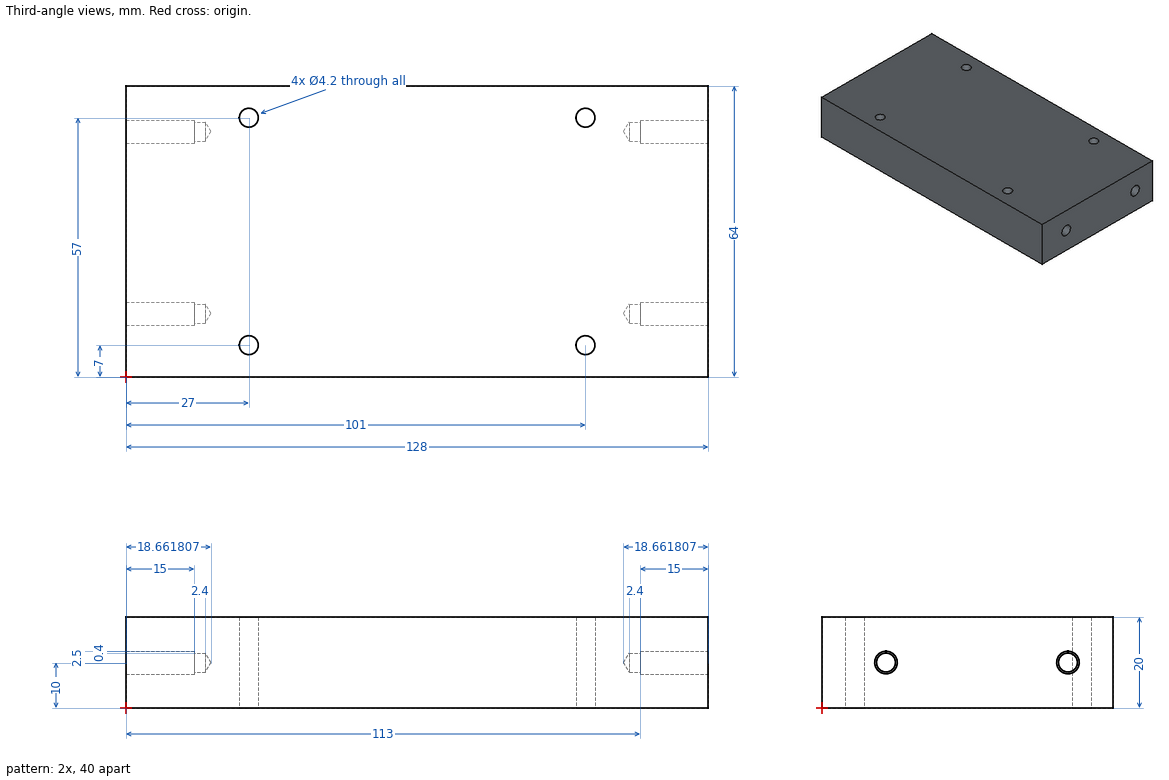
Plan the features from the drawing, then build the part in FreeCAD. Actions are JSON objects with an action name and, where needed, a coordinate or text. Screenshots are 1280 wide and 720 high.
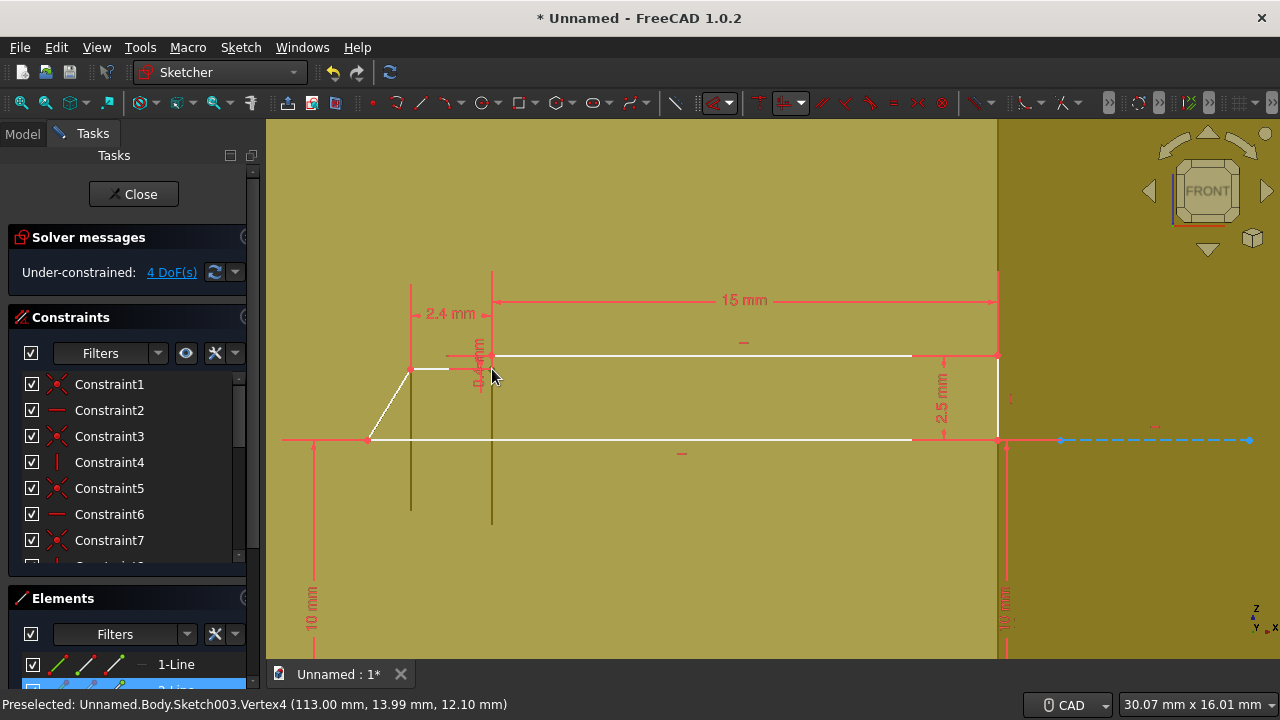
{"action": "key", "text": "l"}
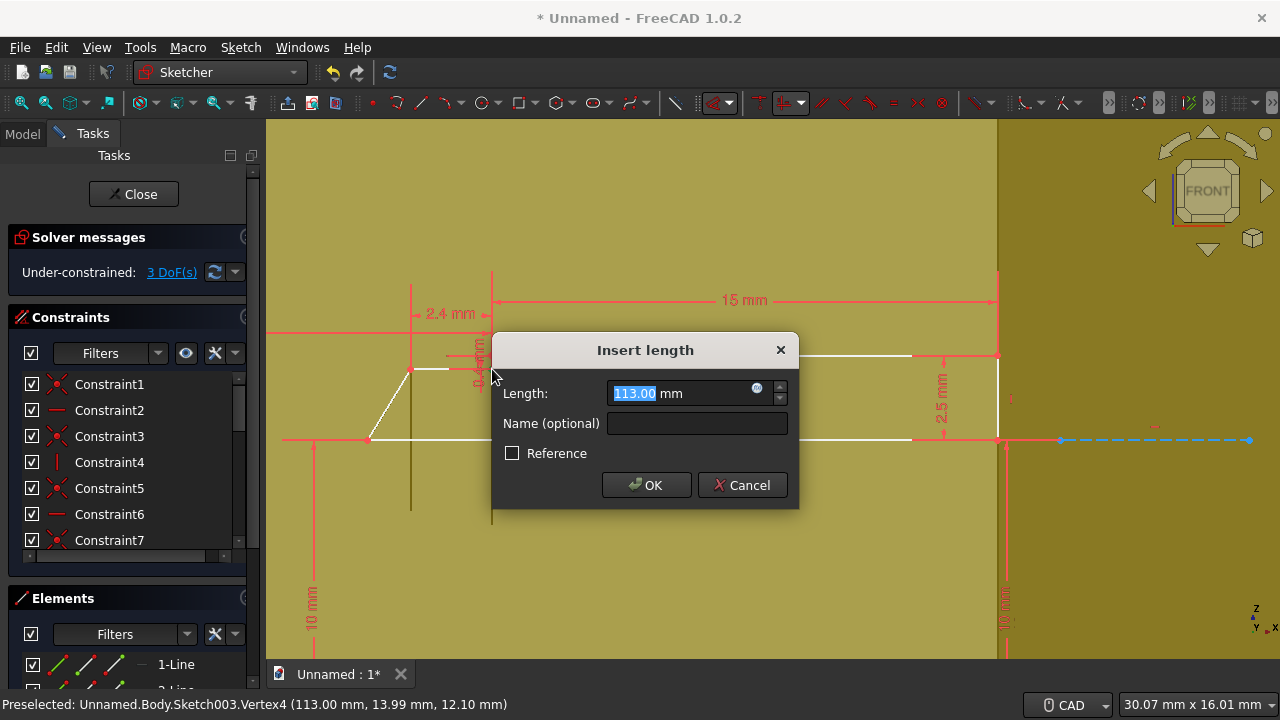
{"action": "type", "text": "113"}
{"action": "key", "text": "Return"}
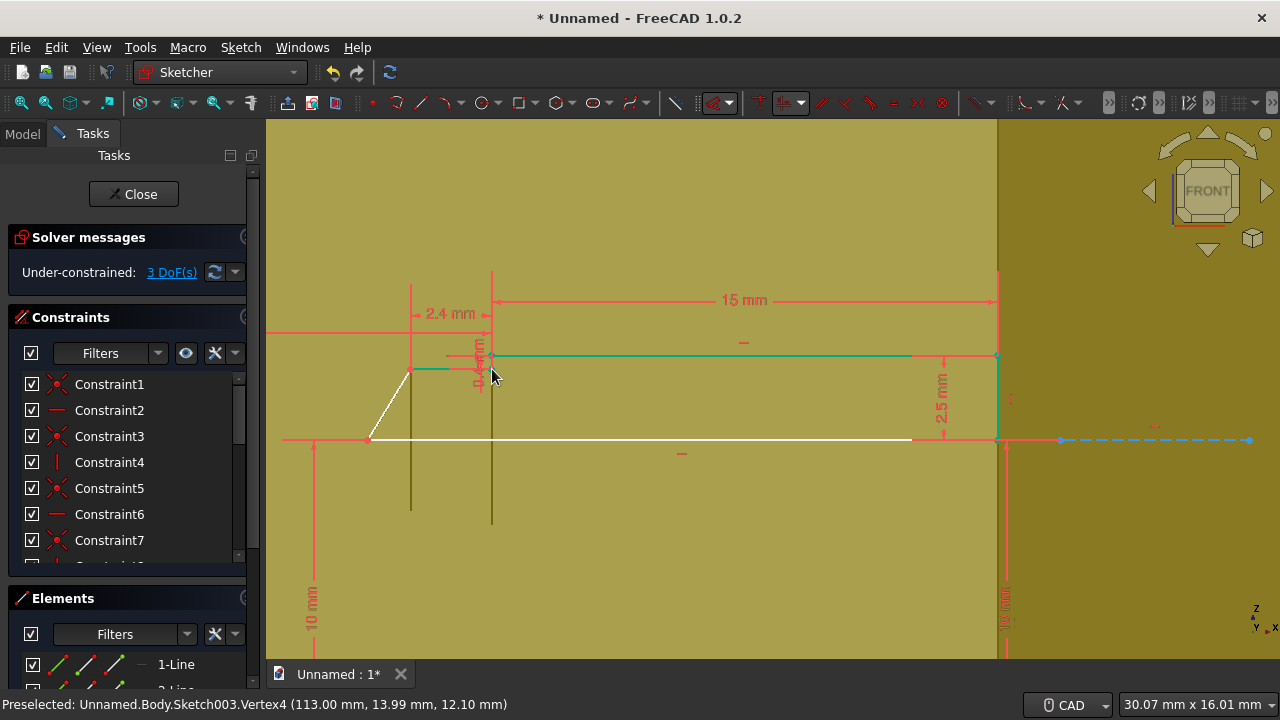
{"action": "left_click", "coordinate": [809, 440]}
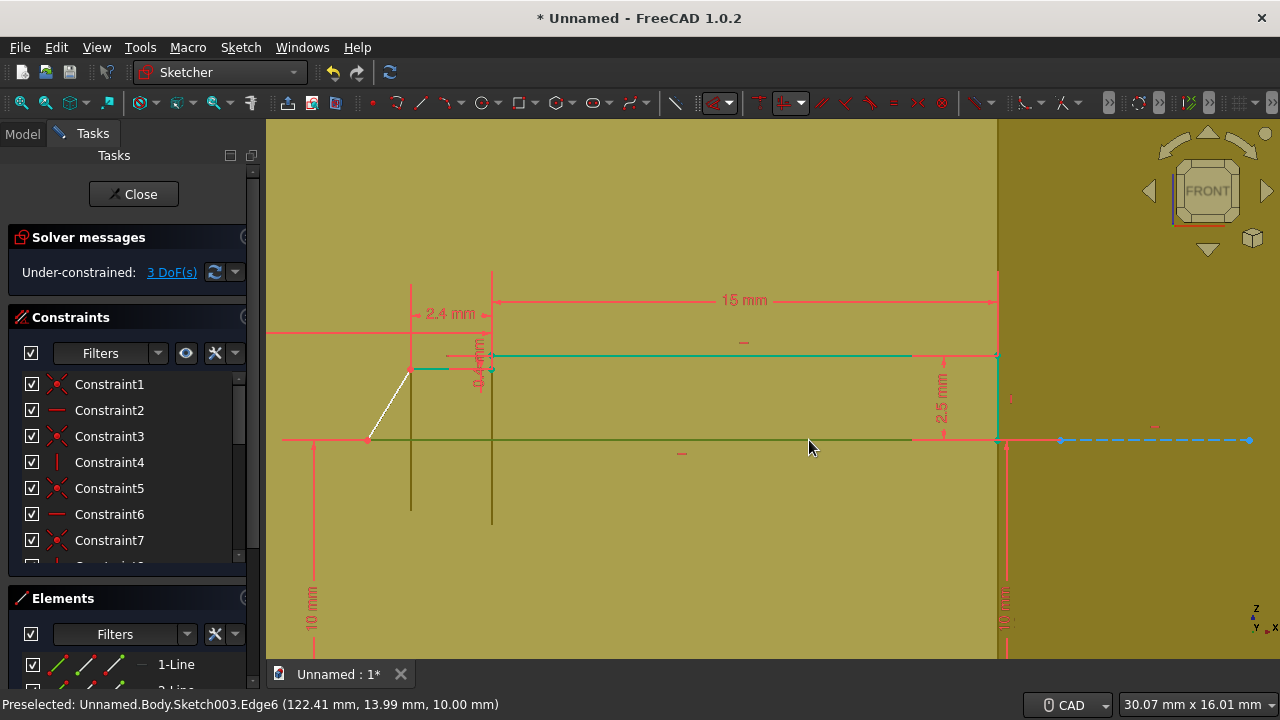
{"action": "left_click", "coordinate": [732, 104]}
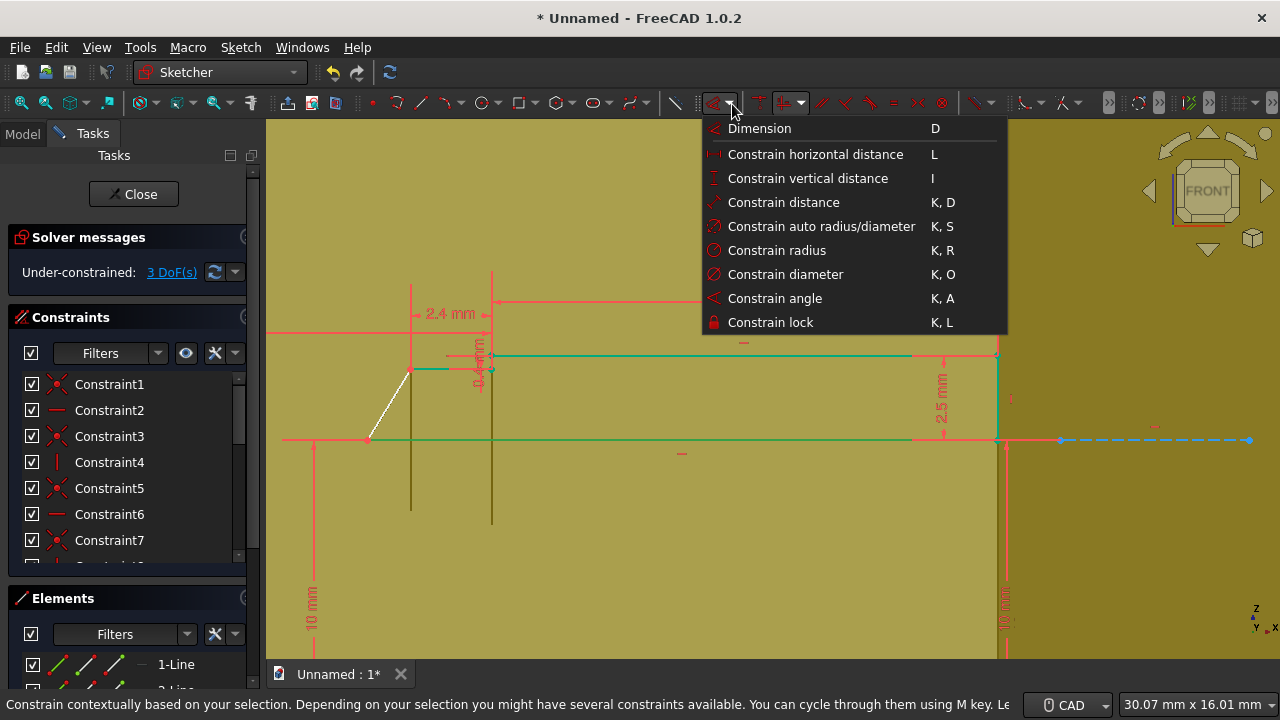
{"action": "left_click", "coordinate": [855, 154]}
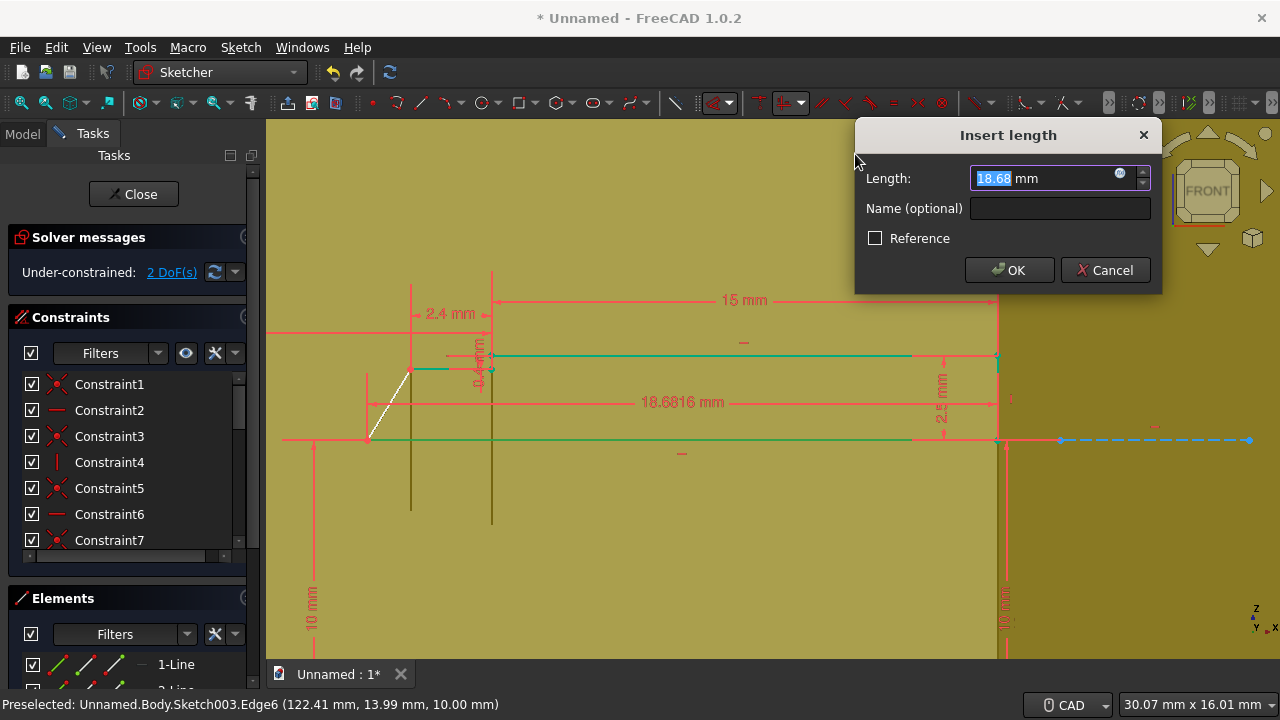
{"action": "type", "text": "18.661807"}
{"action": "key", "text": "Return"}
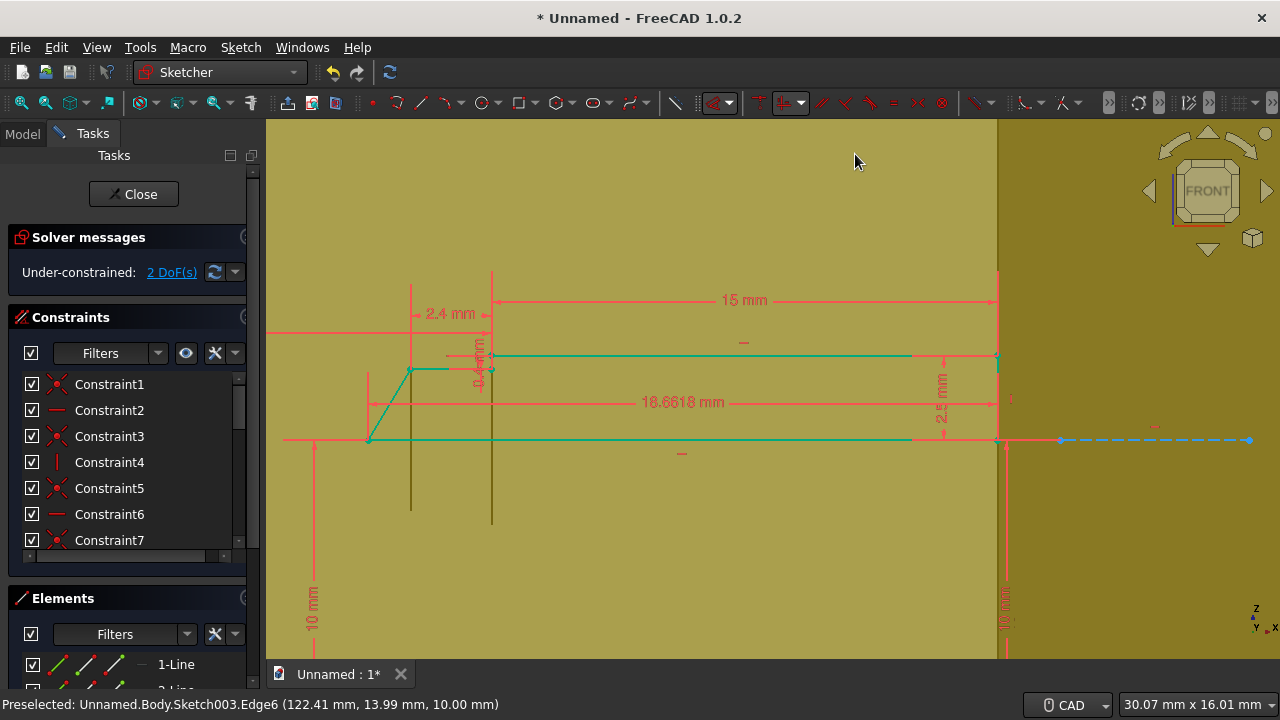
{"action": "left_click", "coordinate": [134, 194]}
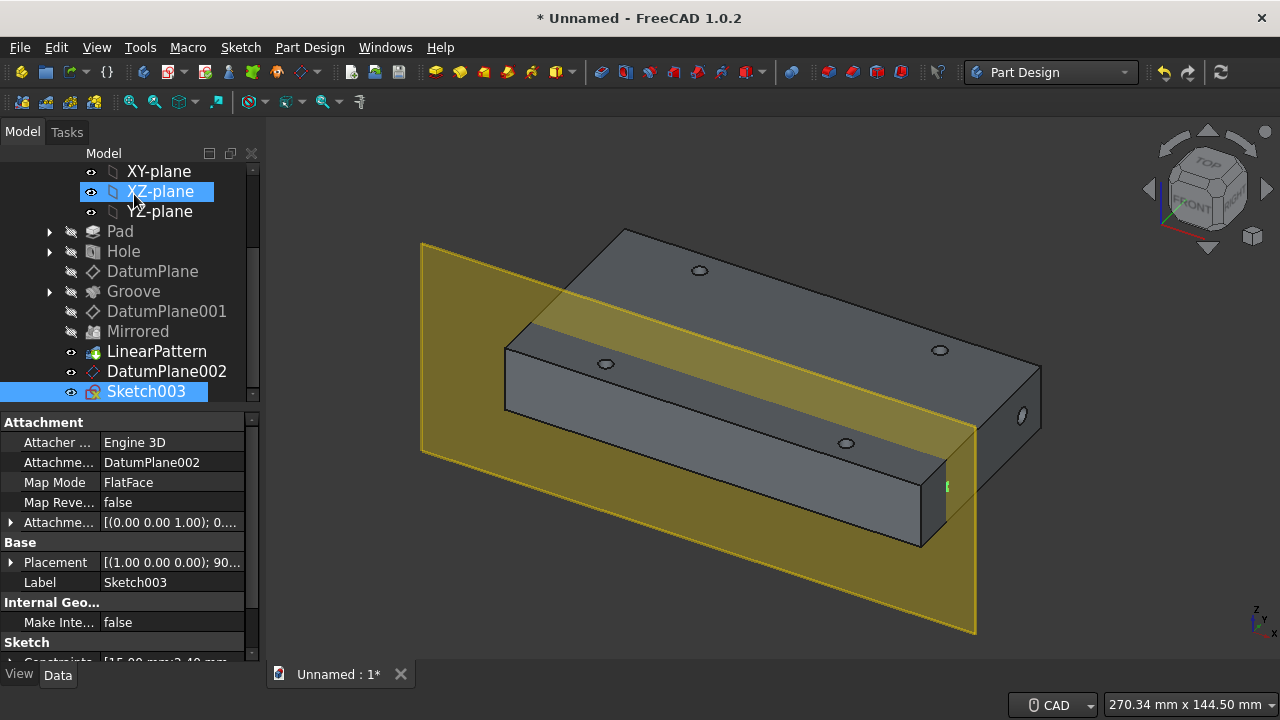
{"action": "left_click", "coordinate": [650, 72]}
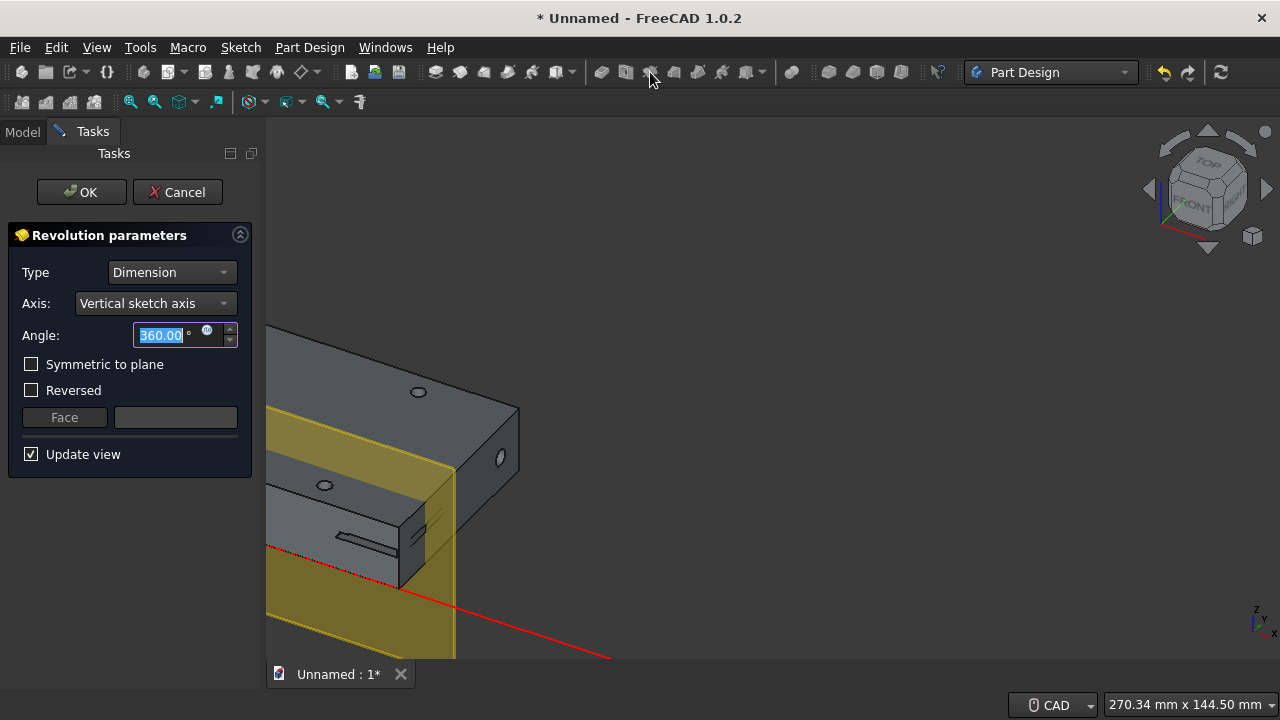
{"action": "left_click", "coordinate": [156, 304]}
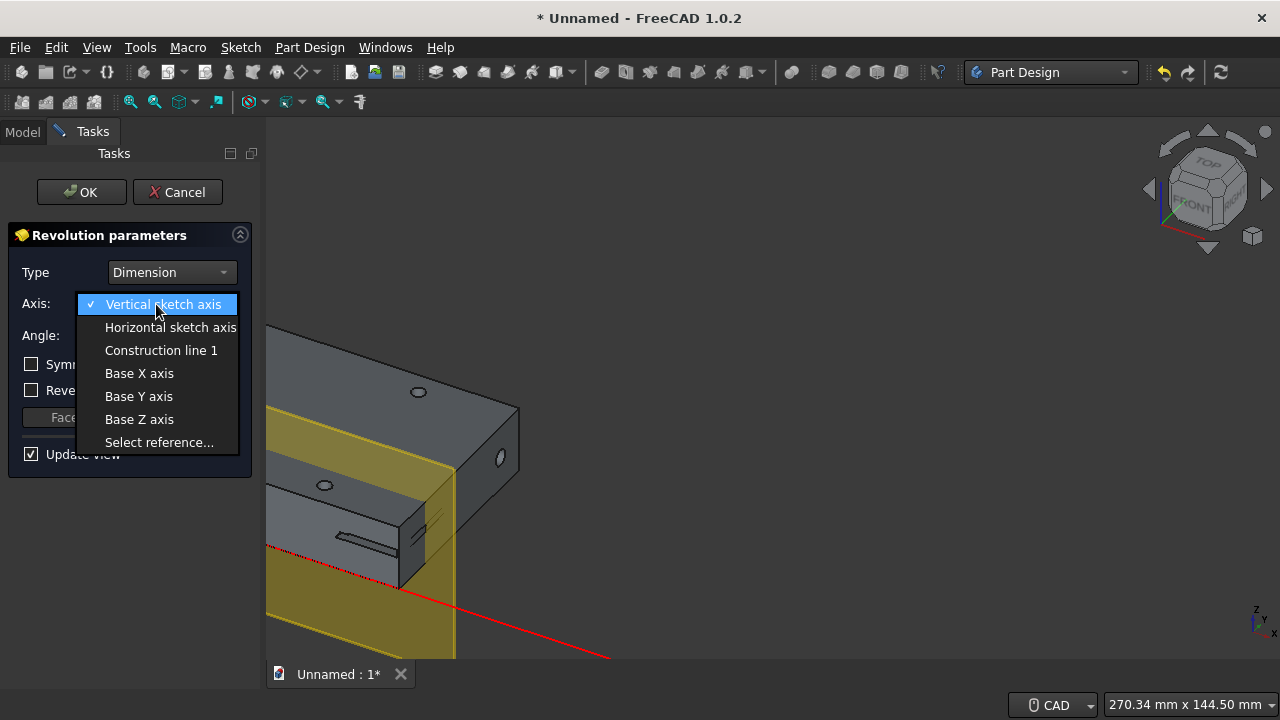
{"action": "left_click", "coordinate": [156, 350]}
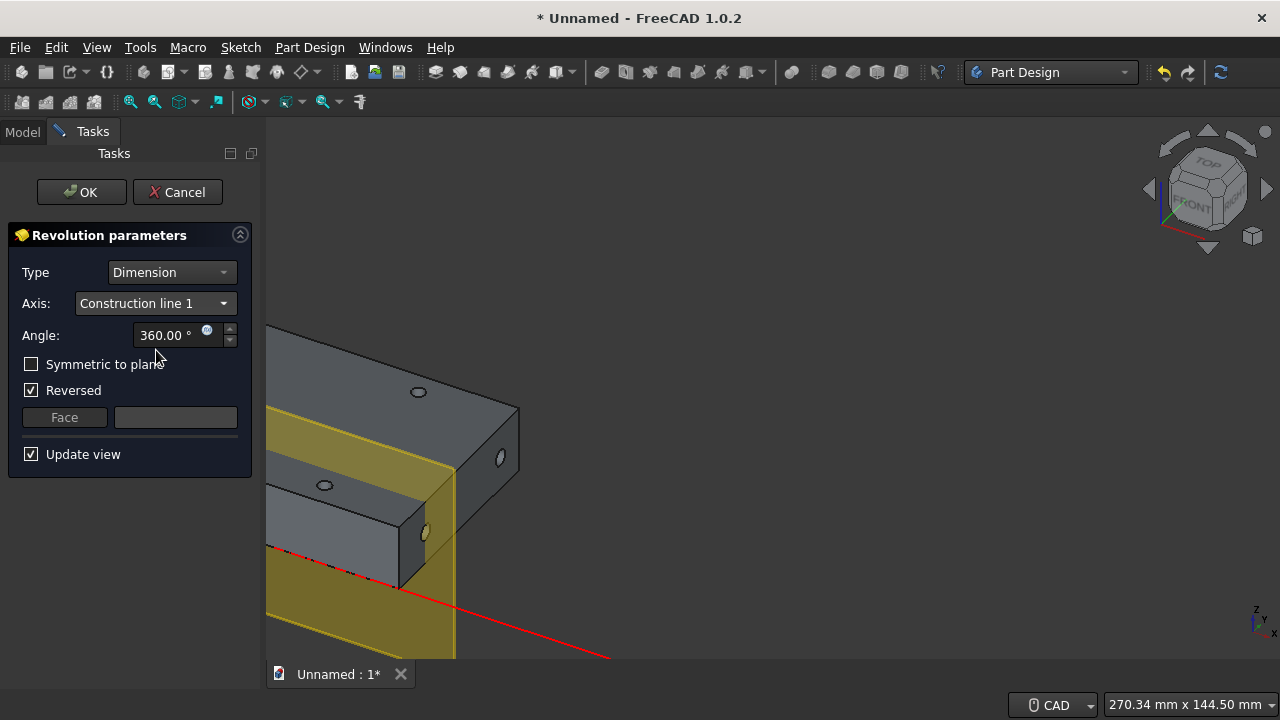
{"action": "left_click", "coordinate": [82, 192]}